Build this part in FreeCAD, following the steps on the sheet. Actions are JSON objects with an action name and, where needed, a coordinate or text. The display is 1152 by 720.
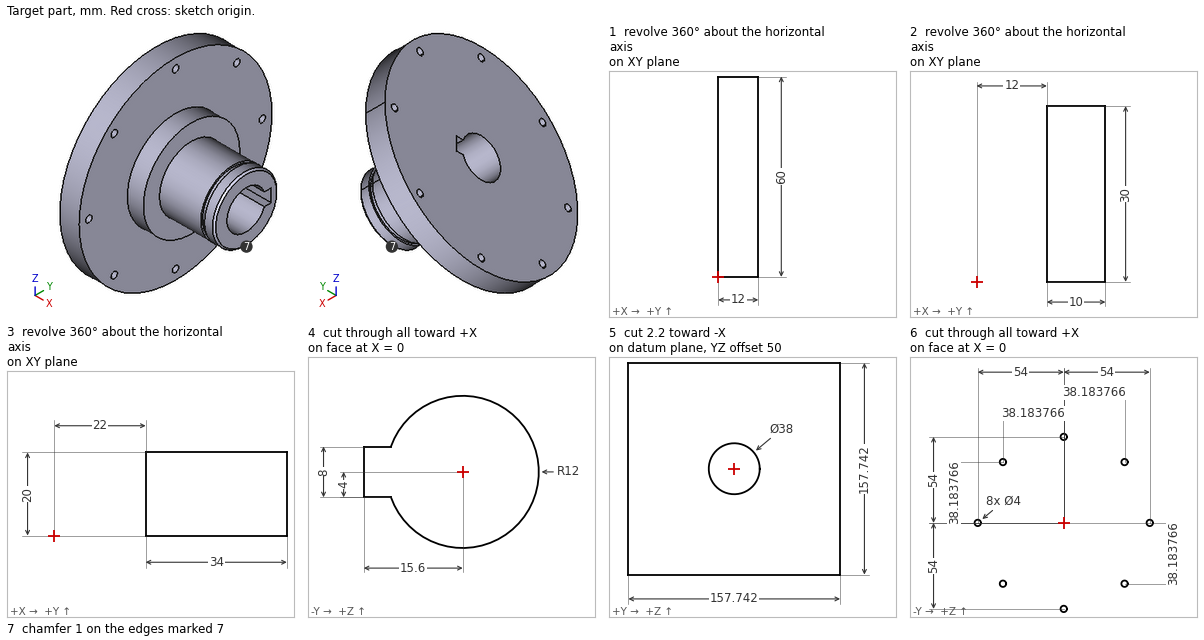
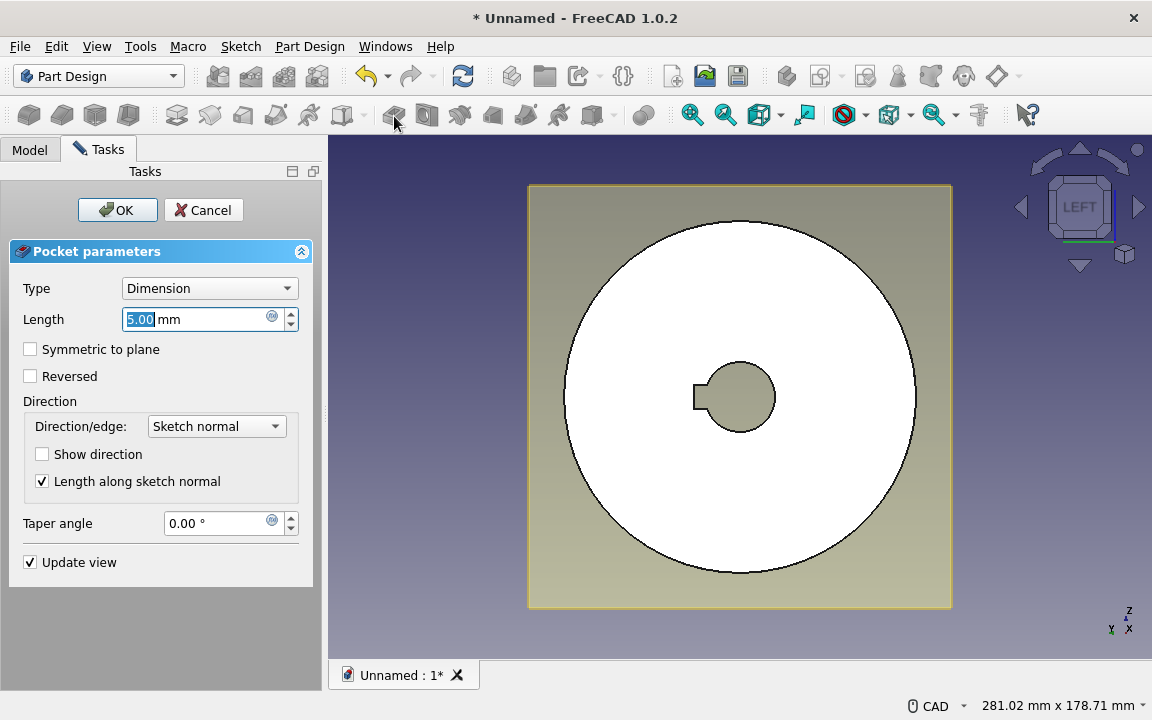
{"action": "type", "text": "2.2"}
{"action": "key", "text": "Tab"}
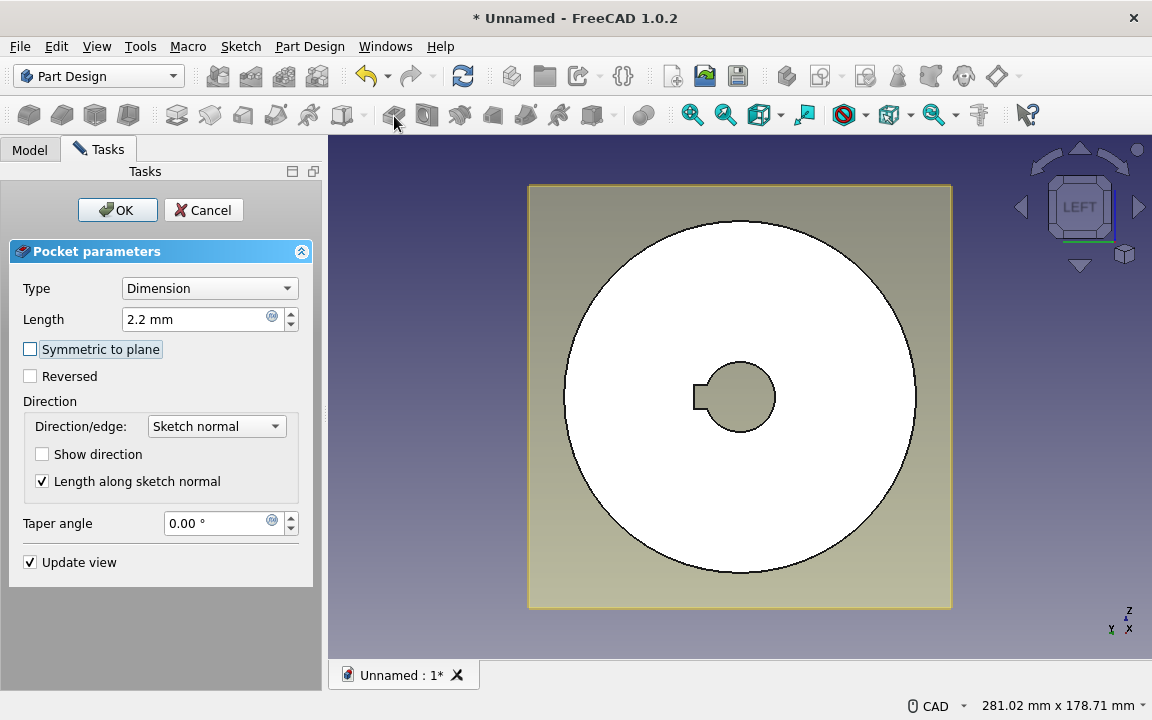
{"action": "left_click", "coordinate": [118, 210]}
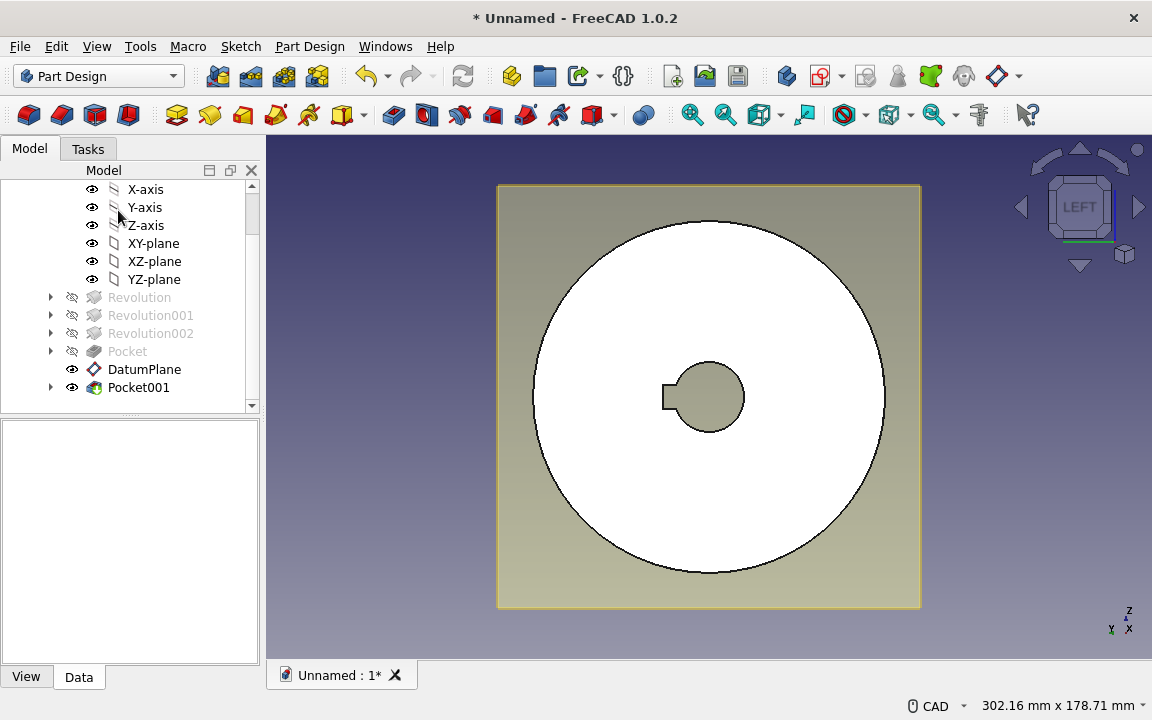
{"action": "left_click", "coordinate": [117, 369]}
{"action": "key", "text": "space"}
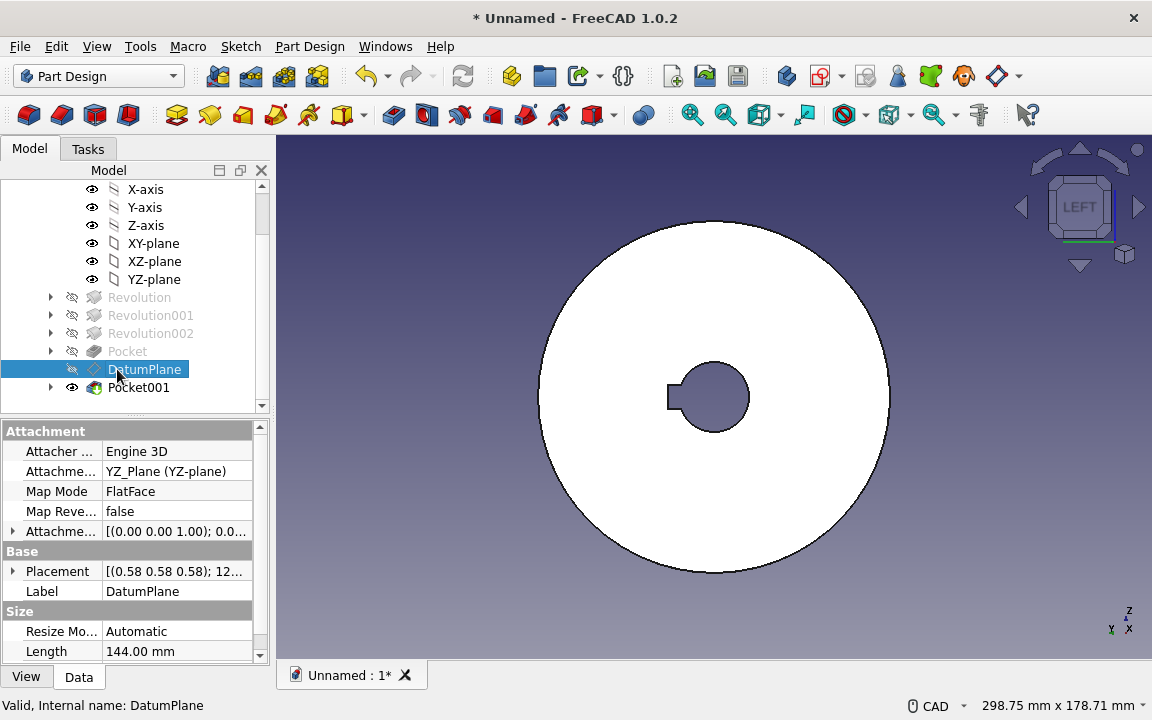
{"action": "left_click", "coordinate": [714, 295]}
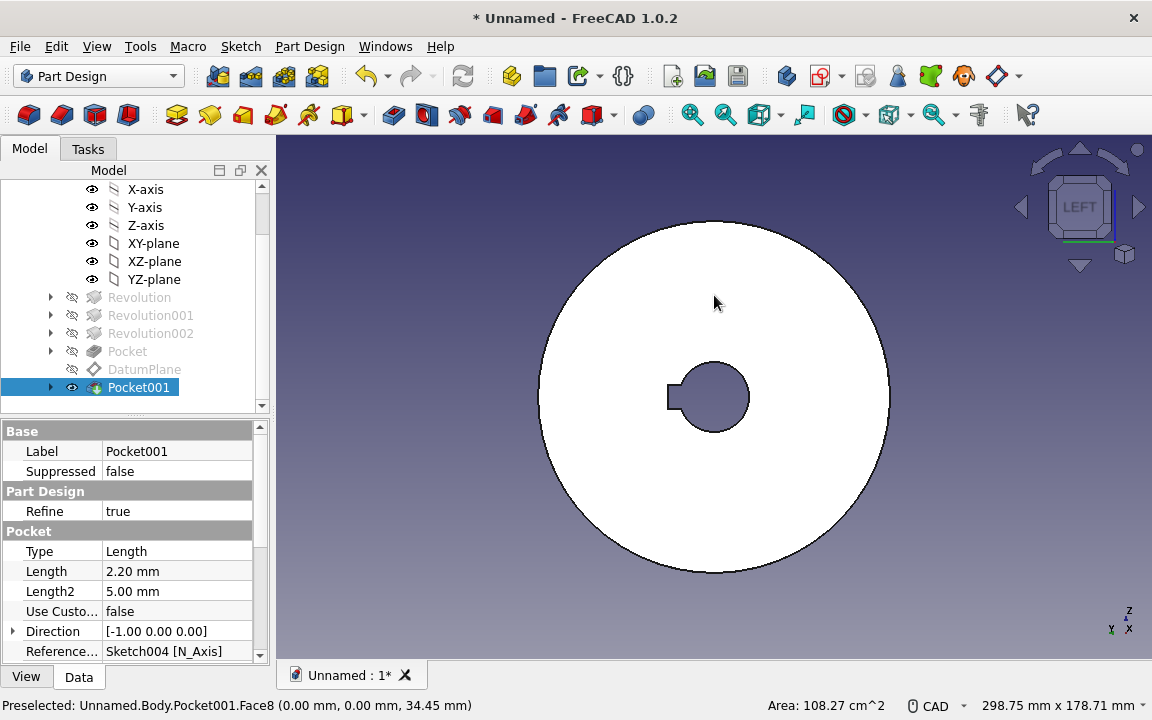
{"action": "left_click", "coordinate": [820, 76]}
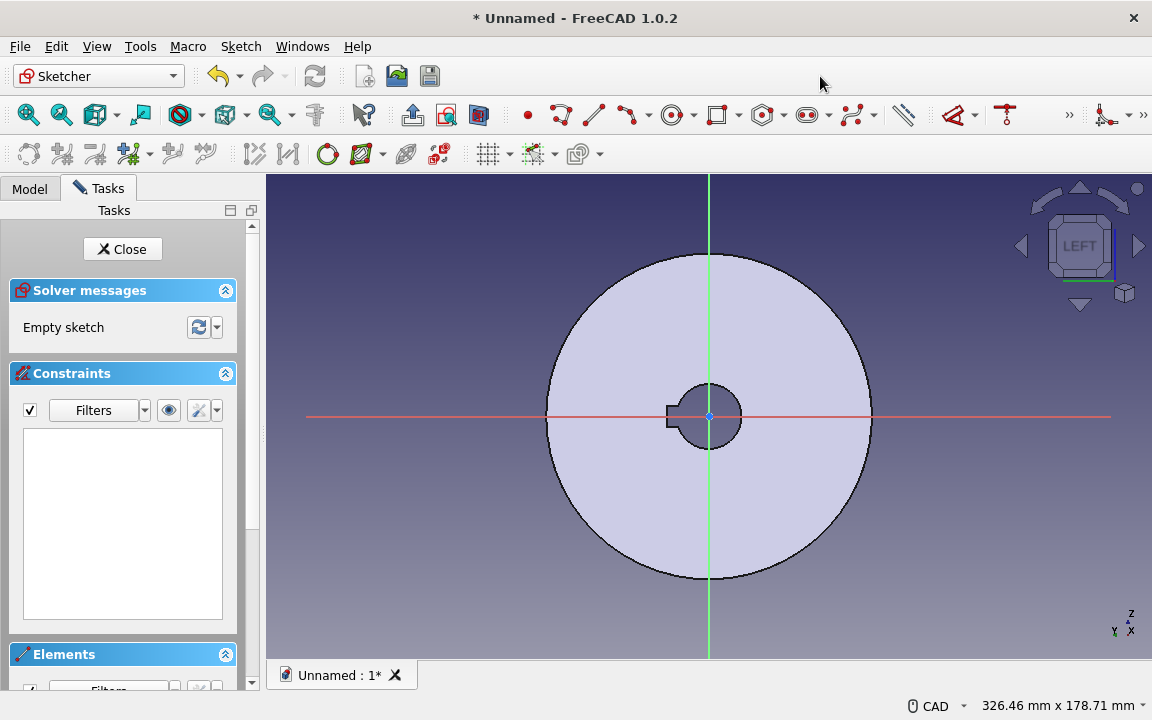
{"action": "left_click", "coordinate": [672, 116]}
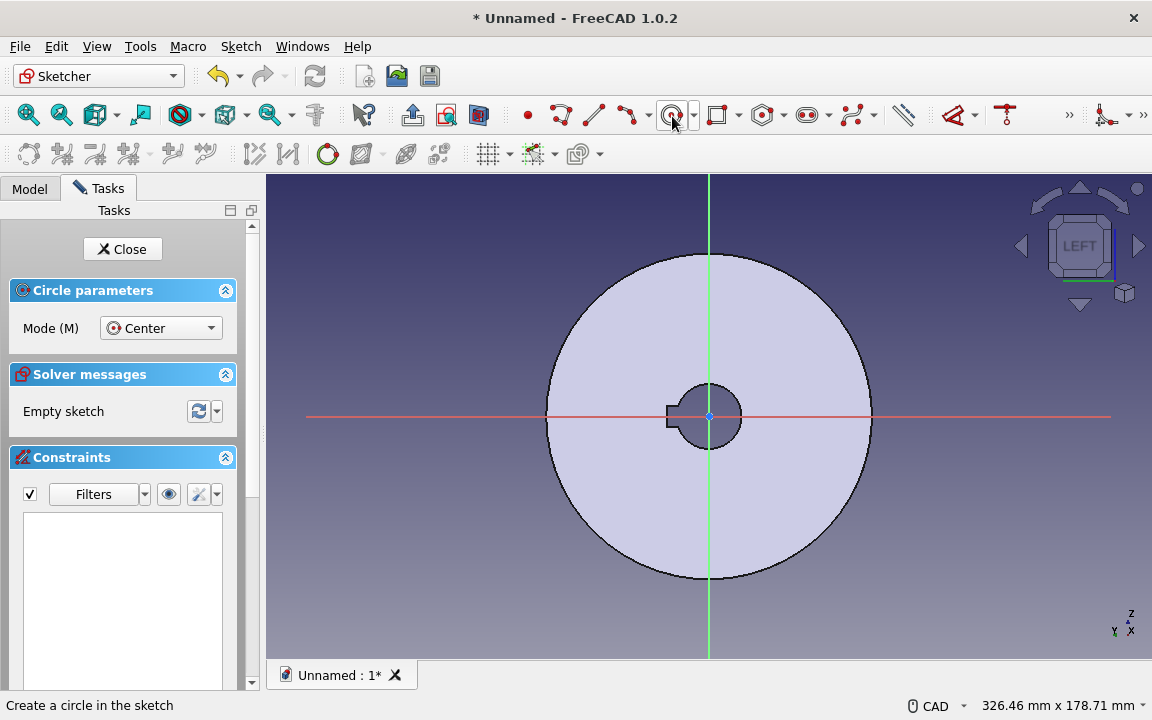
{"action": "scroll", "coordinate": [562, 417], "scroll_direction": "up", "scroll_amount": 8}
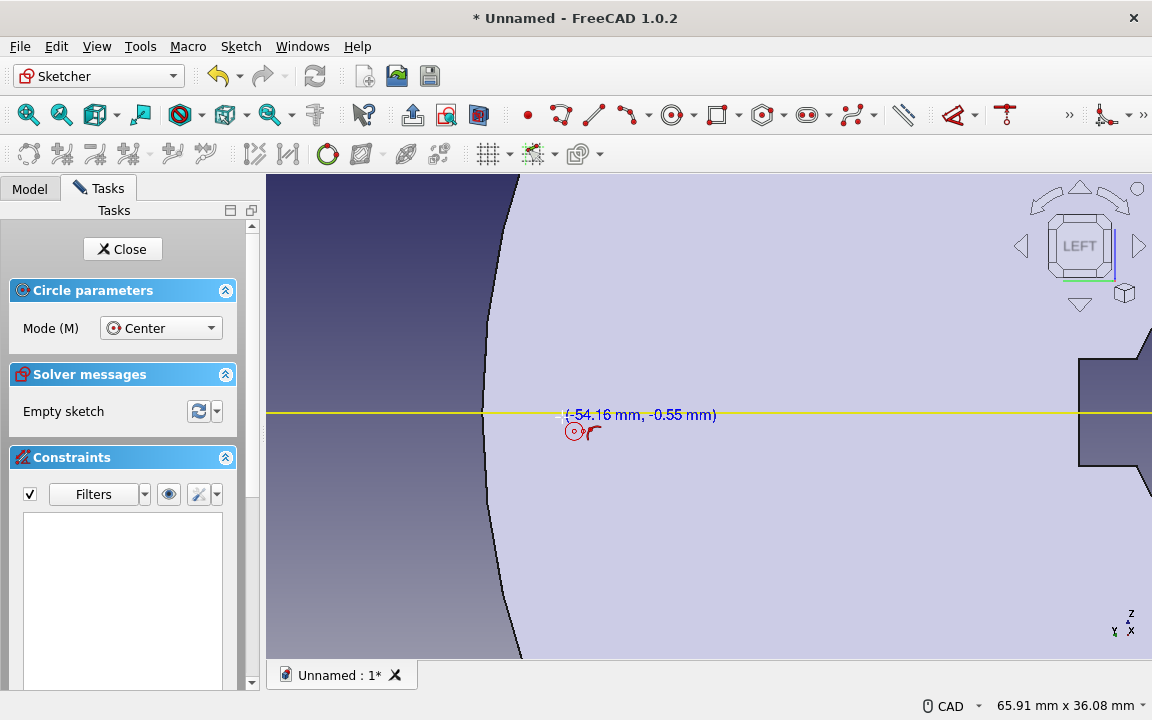
{"action": "scroll", "coordinate": [477, 418], "scroll_direction": "down", "scroll_amount": 8}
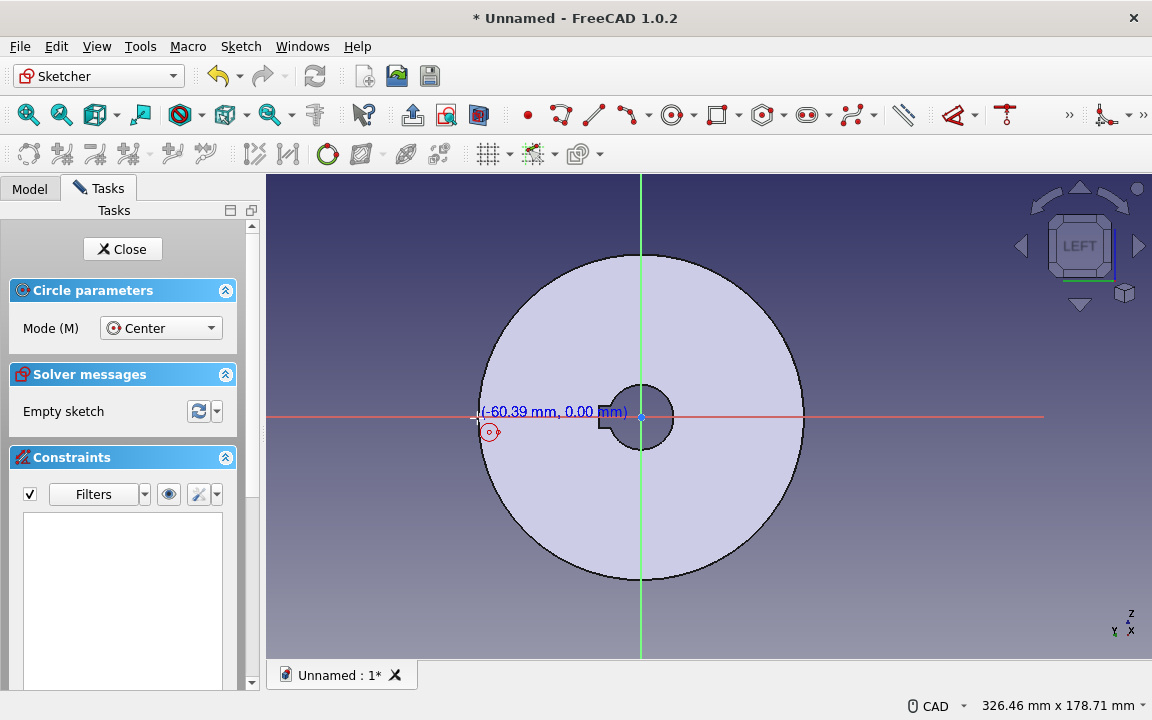
{"action": "left_click", "coordinate": [495, 417]}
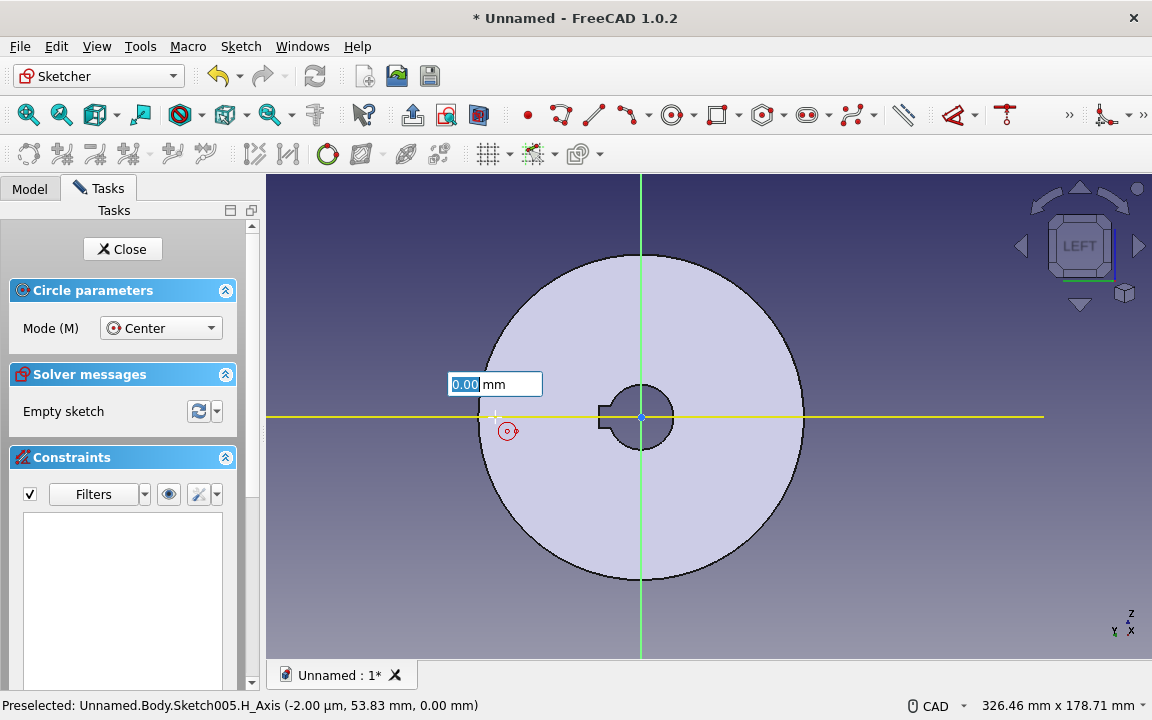
{"action": "scroll", "coordinate": [496, 412], "scroll_direction": "up", "scroll_amount": 6}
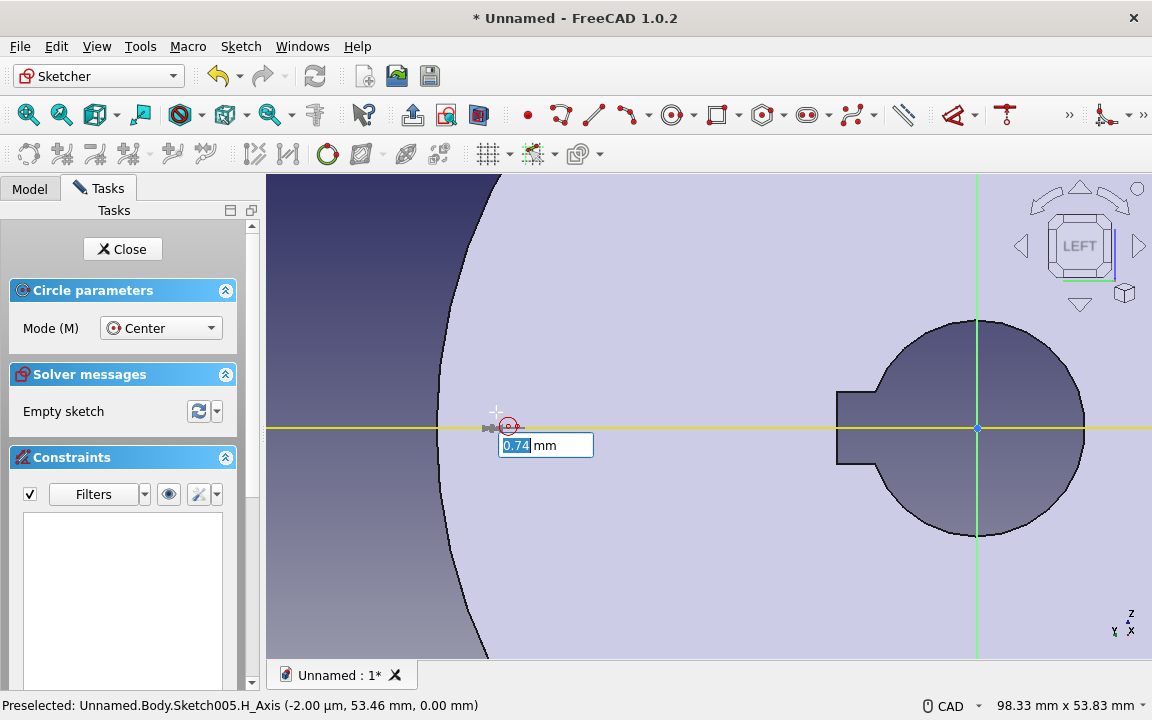
{"action": "left_click", "coordinate": [497, 412]}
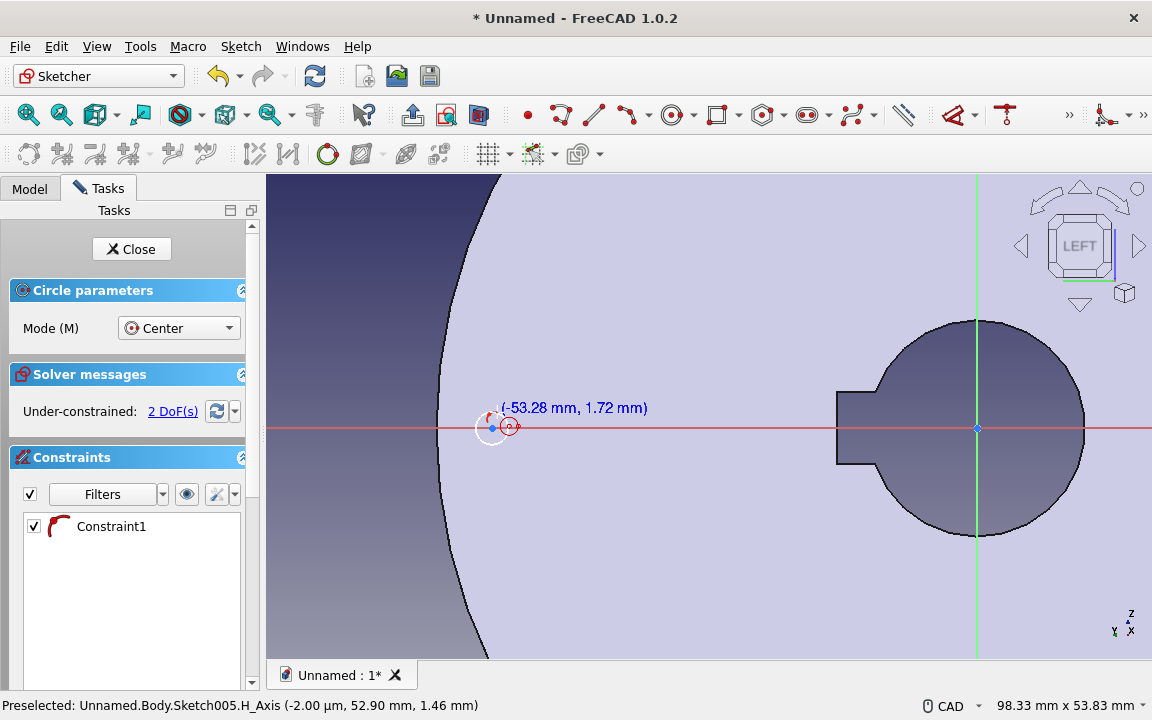
{"action": "scroll", "coordinate": [495, 411], "scroll_direction": "down", "scroll_amount": 6}